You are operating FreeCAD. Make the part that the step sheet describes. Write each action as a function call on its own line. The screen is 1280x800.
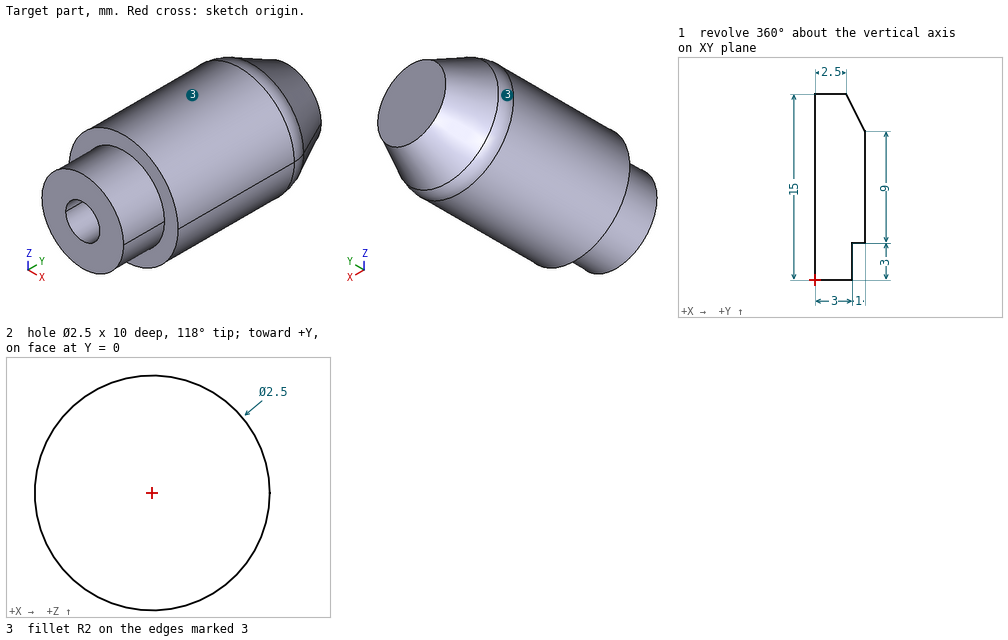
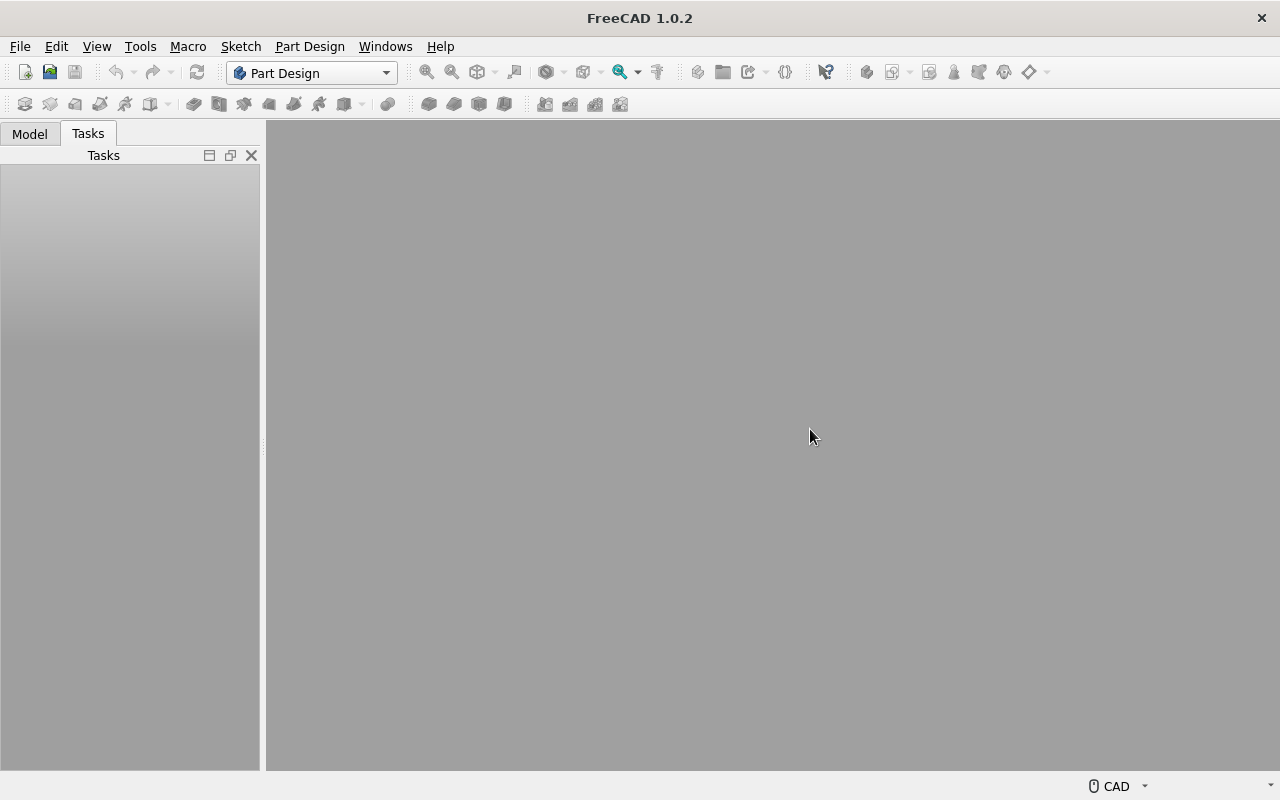
key(ctrl+n)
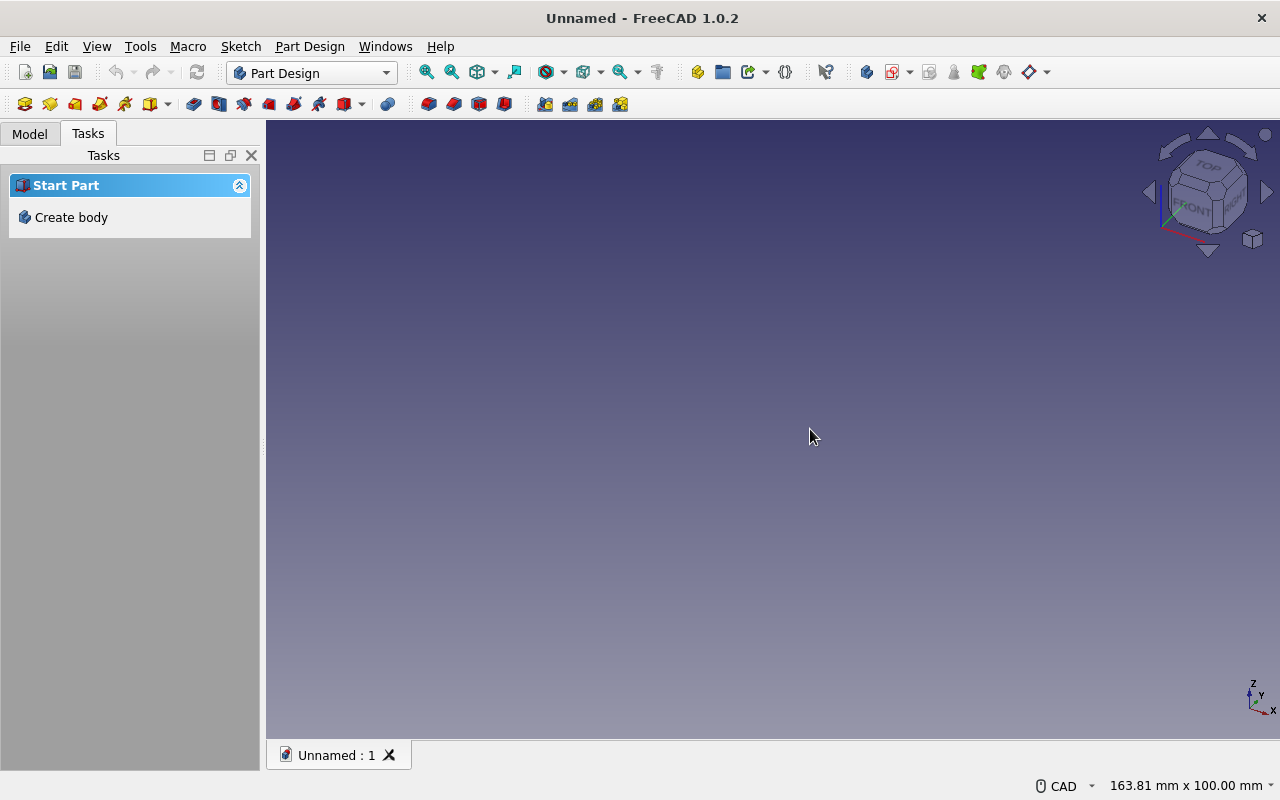
click(892, 72)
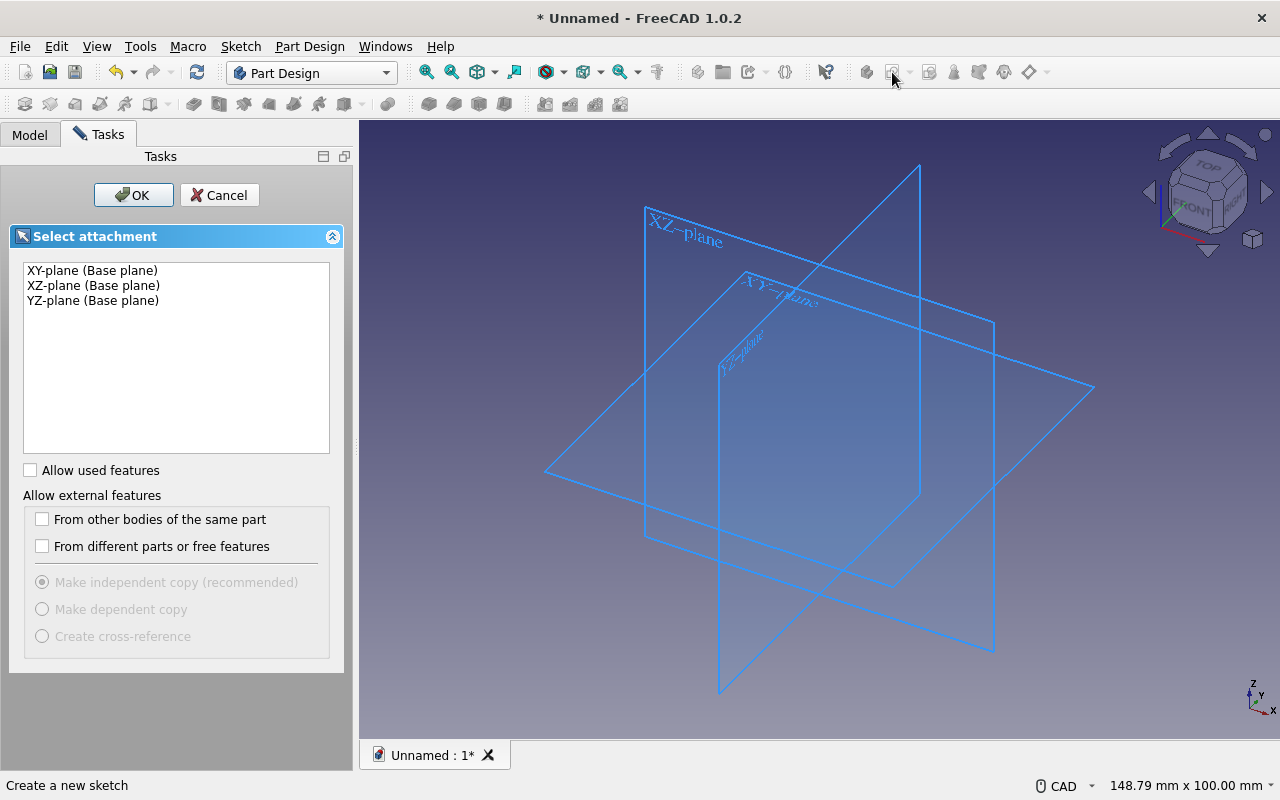
click(84, 270)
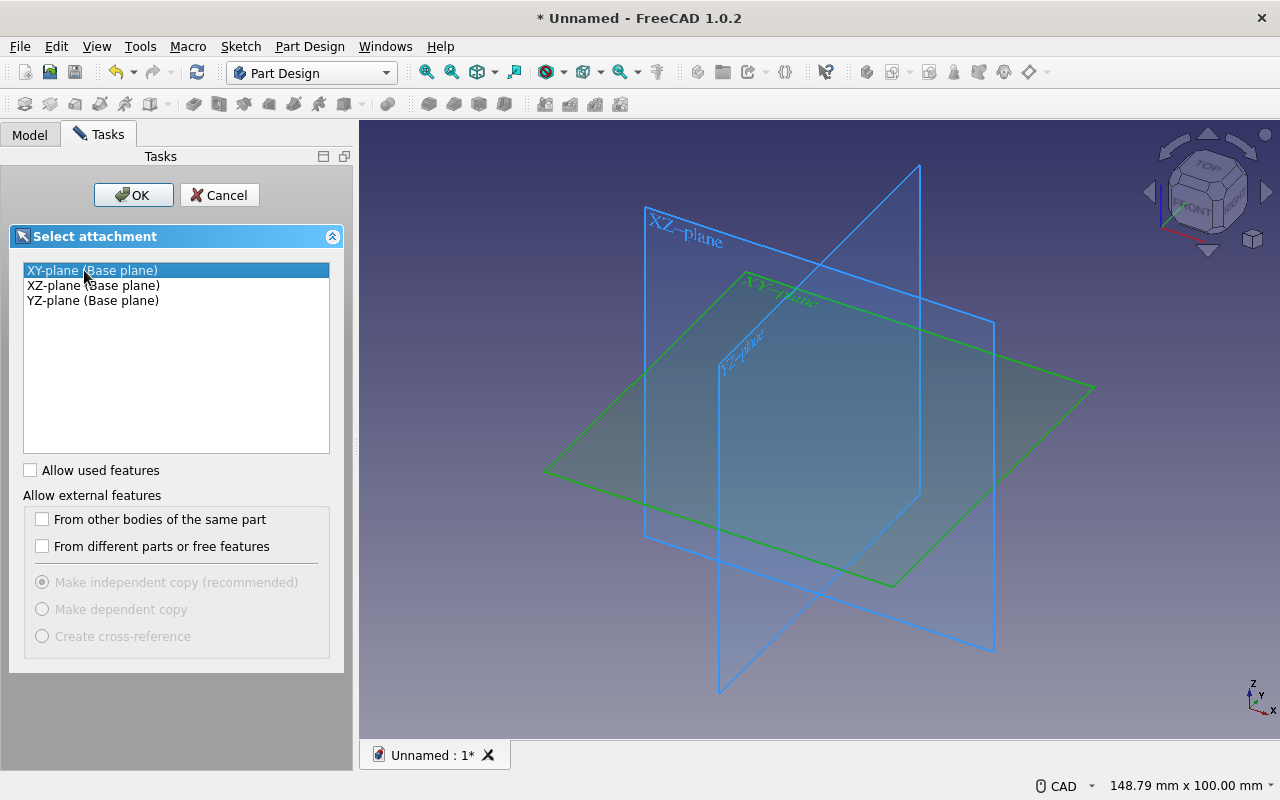
click(134, 195)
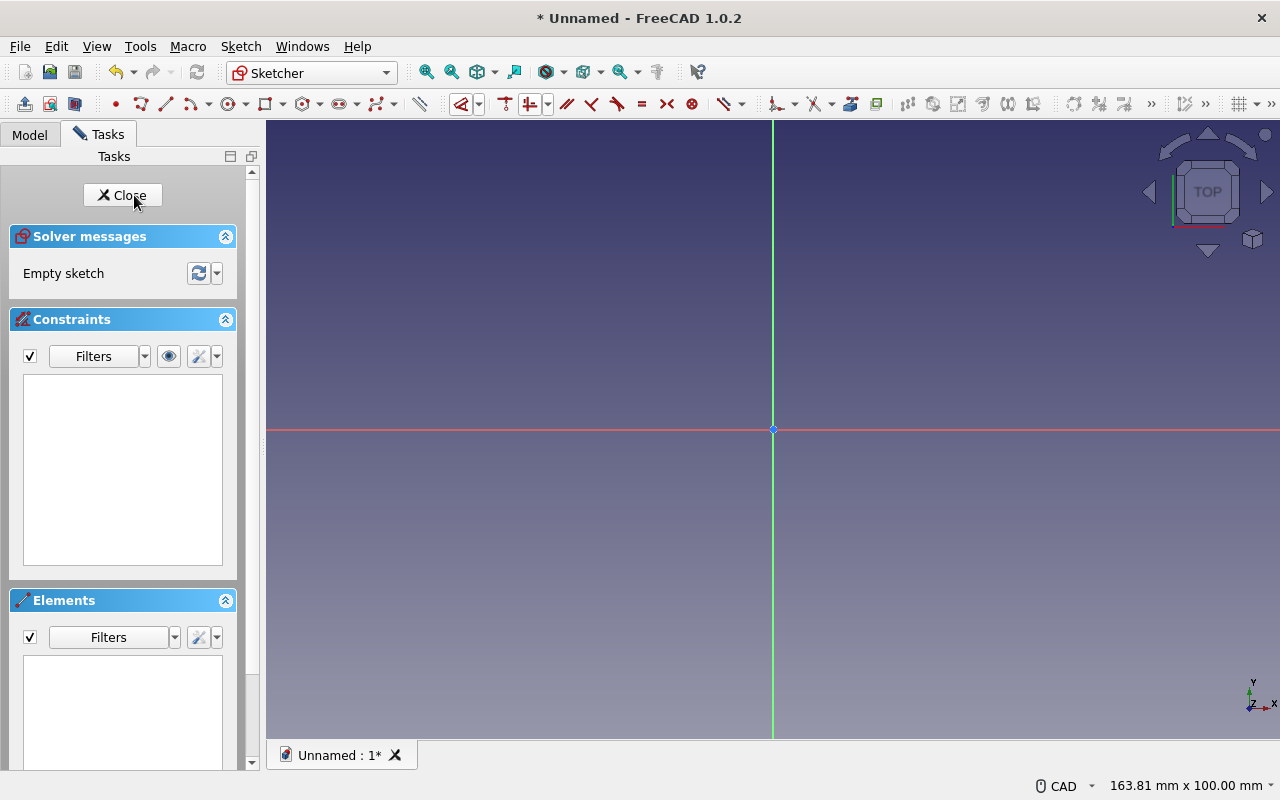
scroll(812, 368, up, 7)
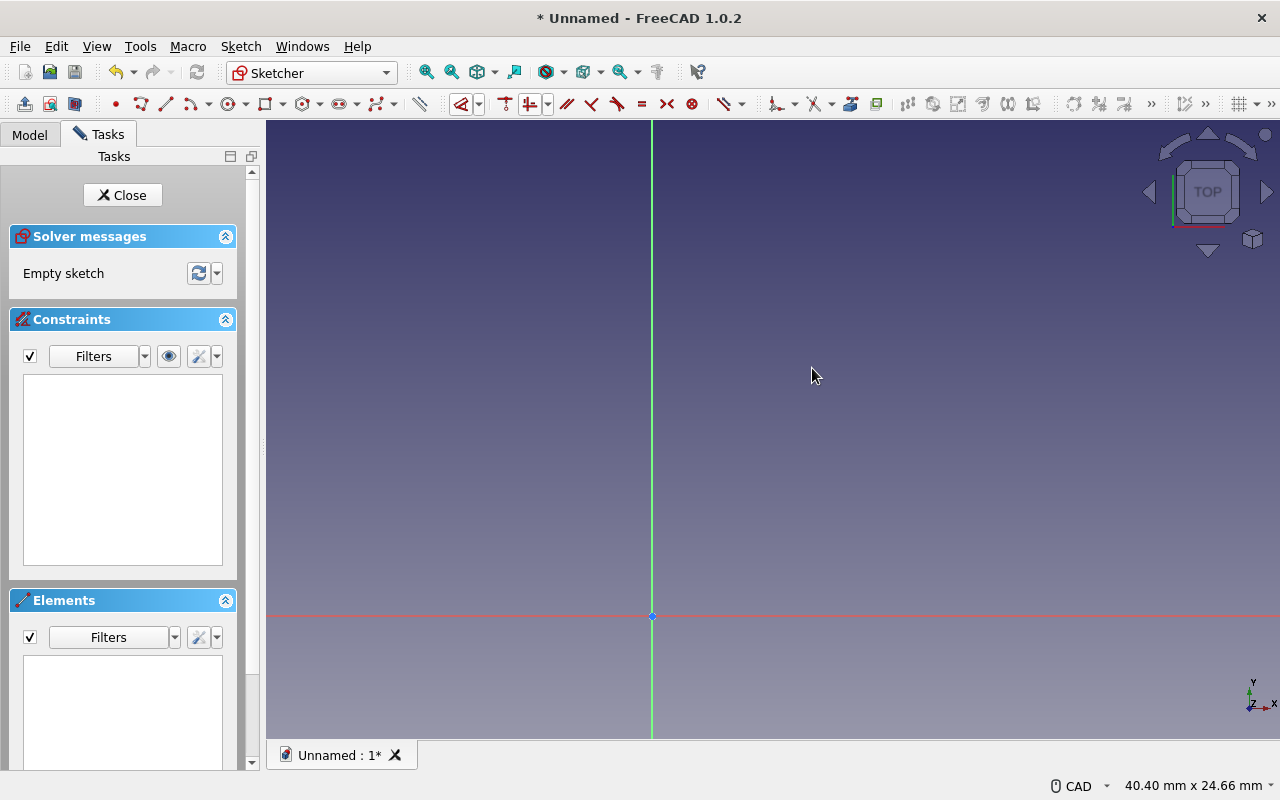
click(141, 104)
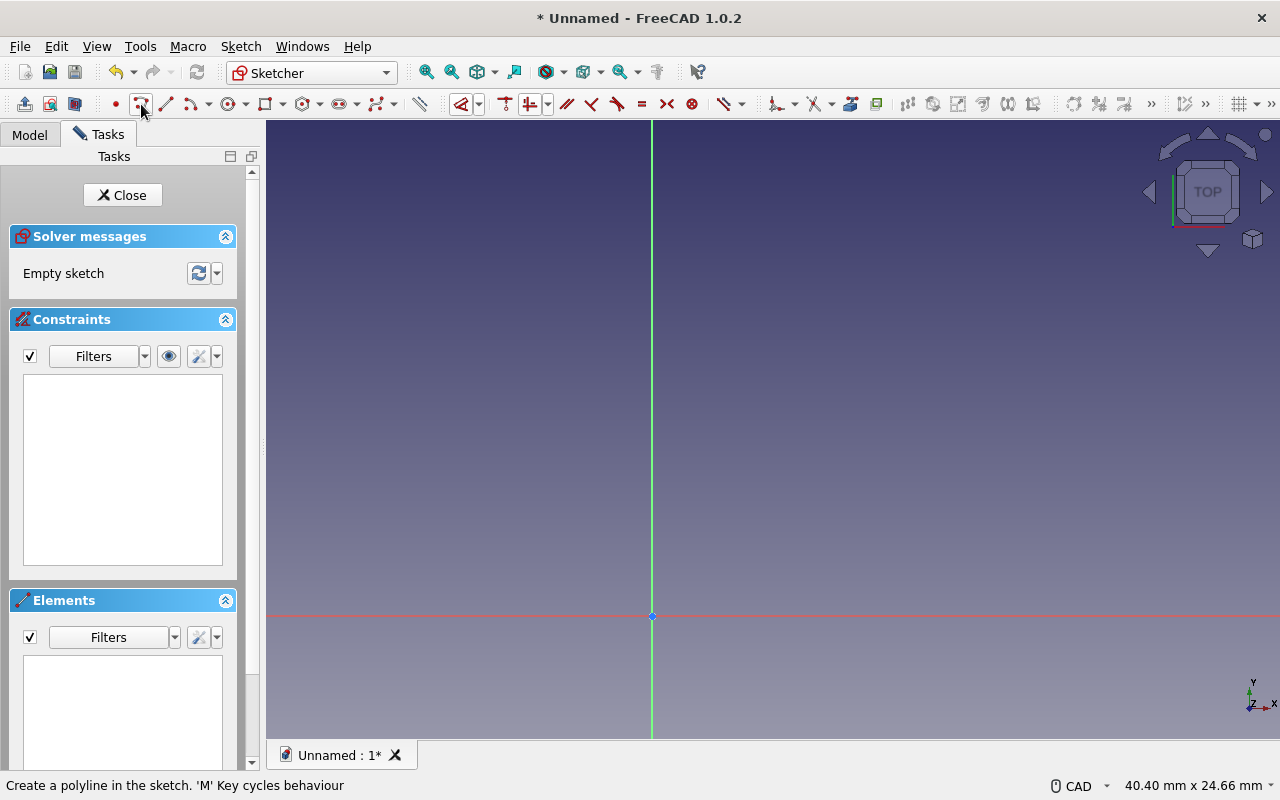
click(652, 616)
click(728, 607)
click(728, 541)
click(753, 541)
click(753, 315)
click(715, 240)
click(661, 240)
click(652, 616)
key(Escape)
key(Escape)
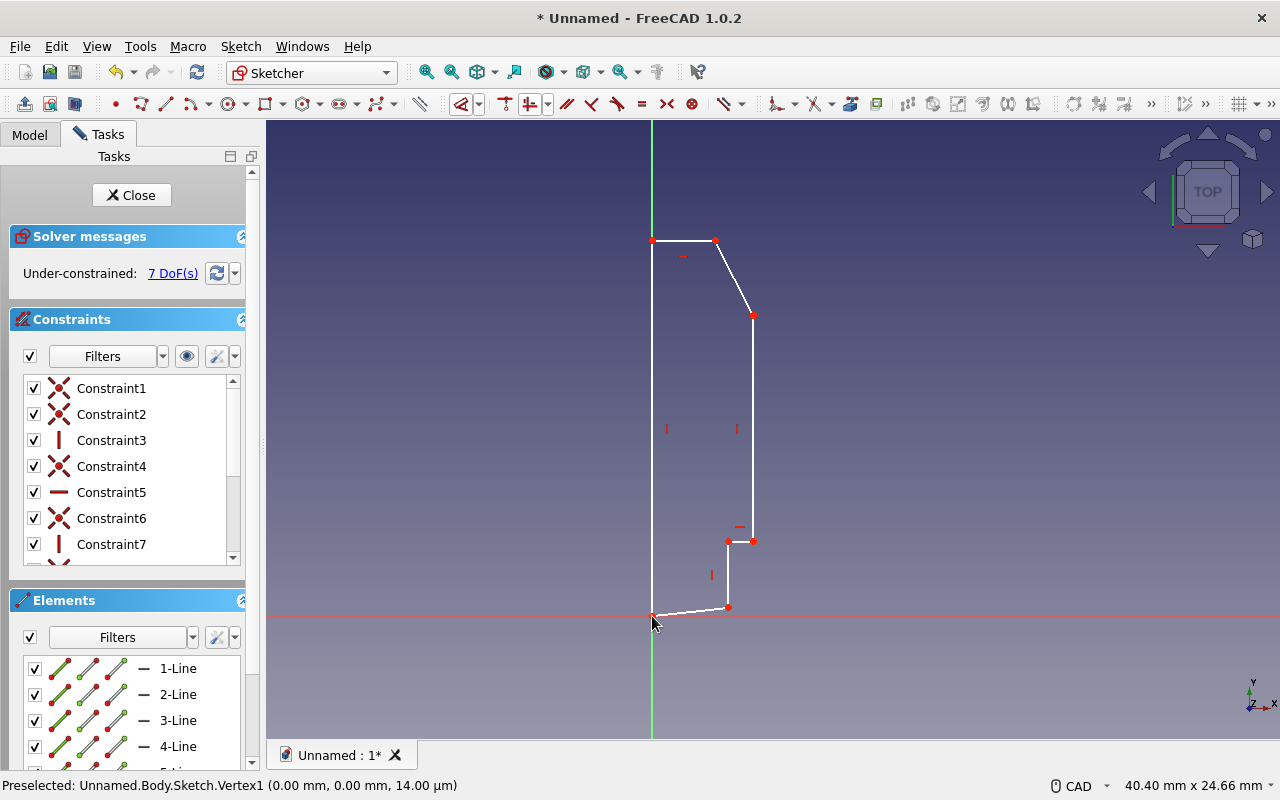
click(675, 614)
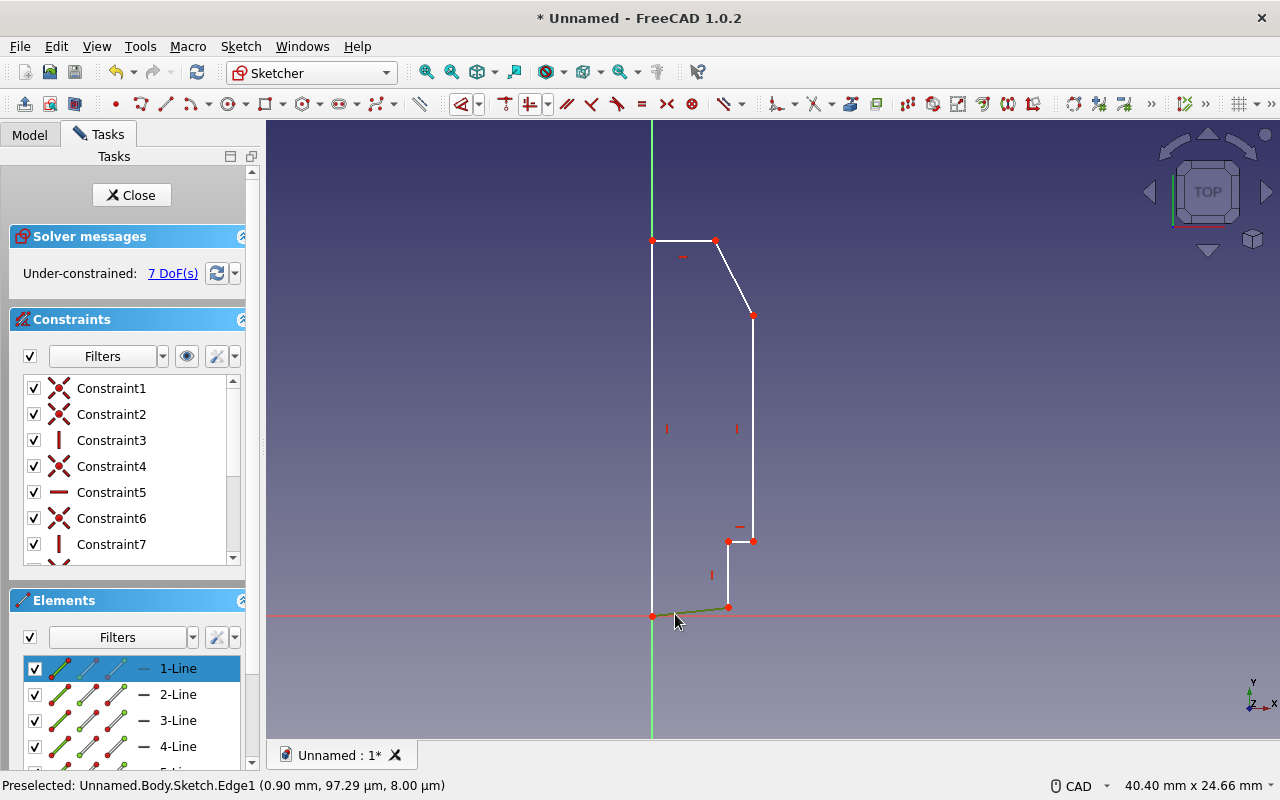
key(h)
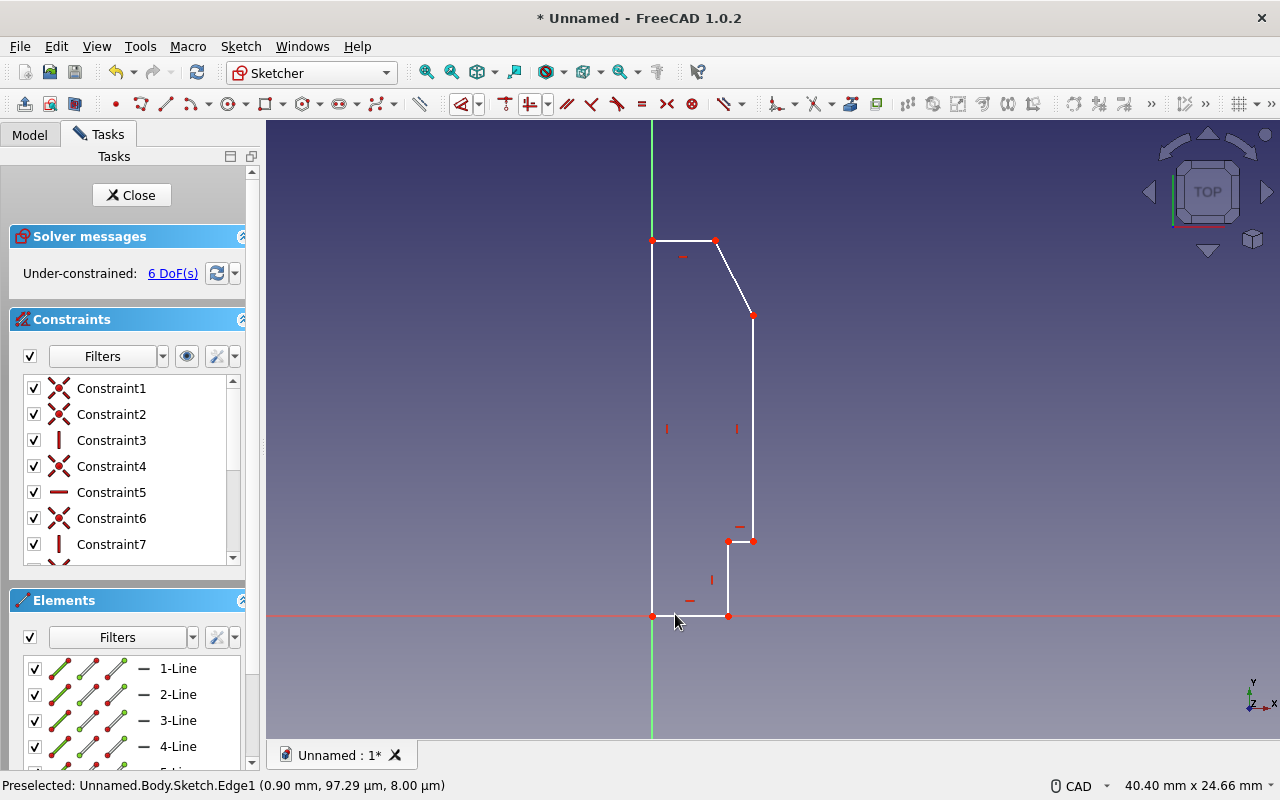
click(460, 104)